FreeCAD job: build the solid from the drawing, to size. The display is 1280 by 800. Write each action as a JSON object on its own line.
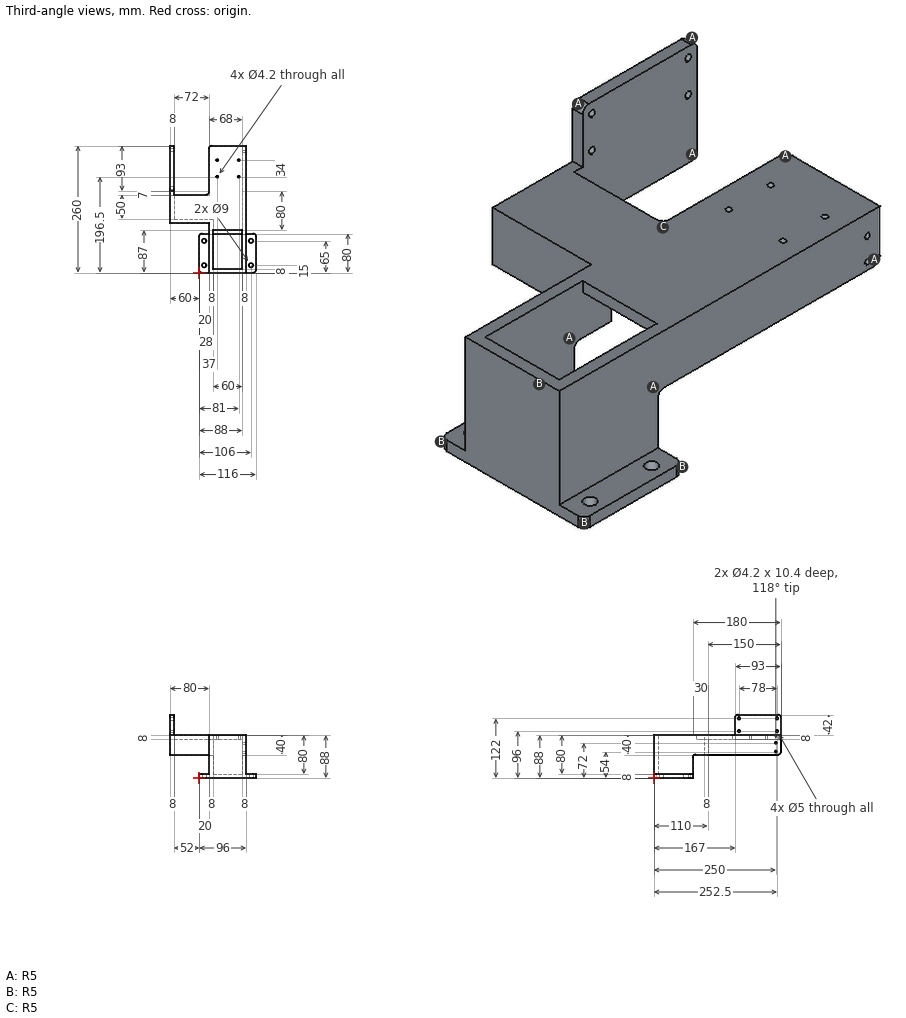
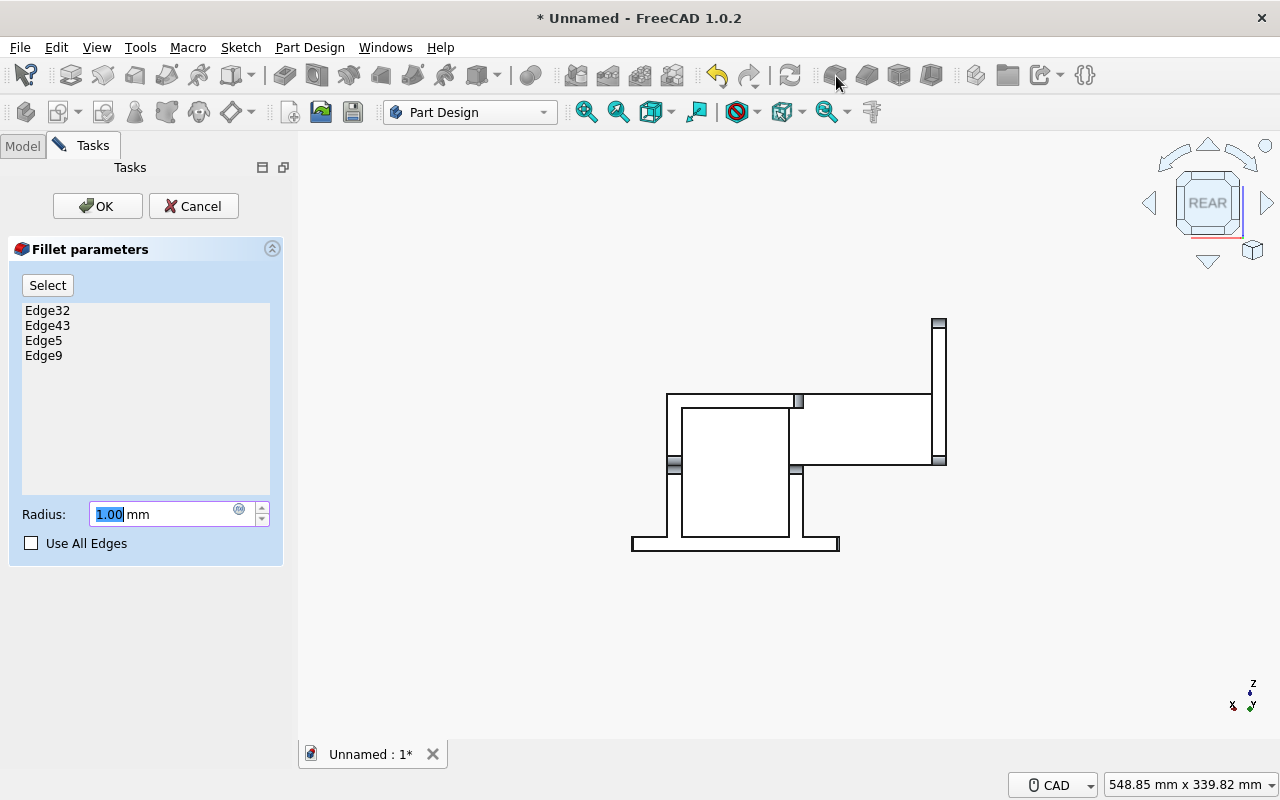
{"action": "type", "text": "5"}
{"action": "key", "text": "Tab"}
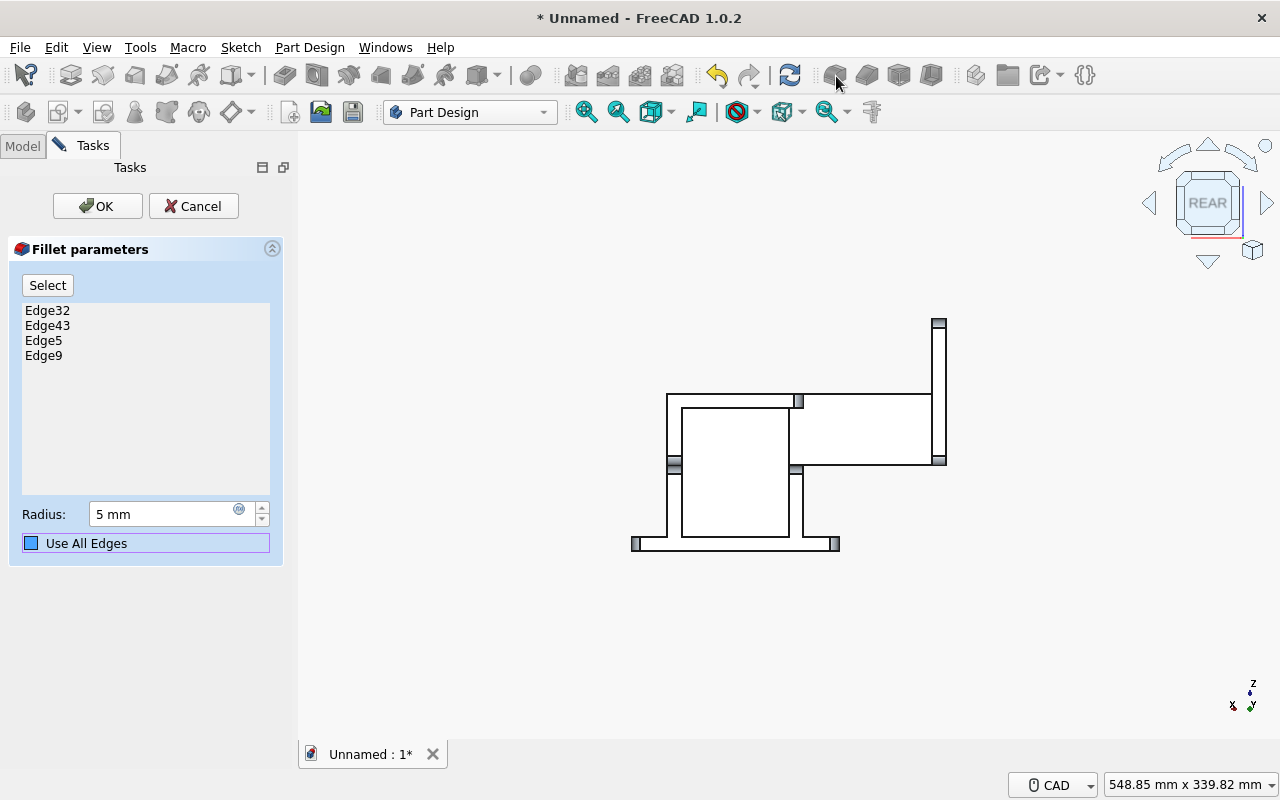
{"action": "left_click", "coordinate": [98, 206]}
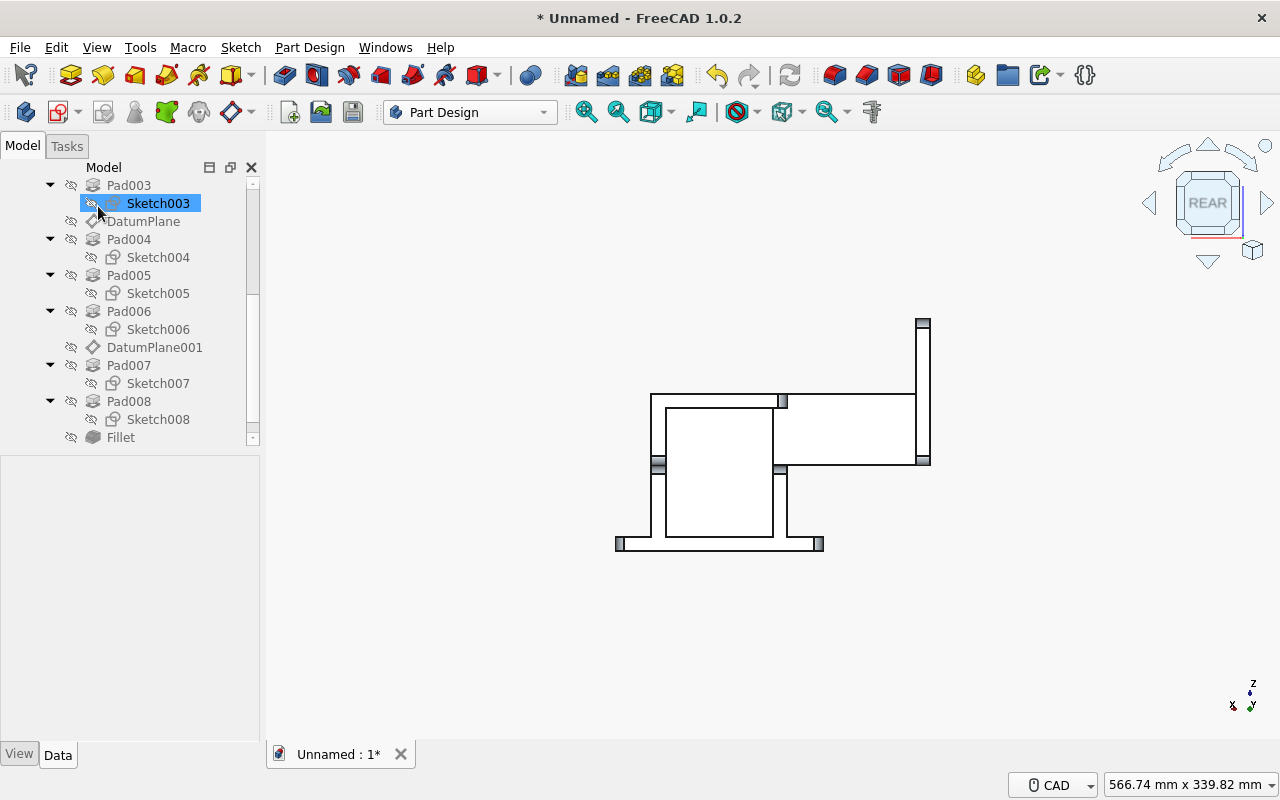
{"action": "left_click", "coordinate": [588, 112]}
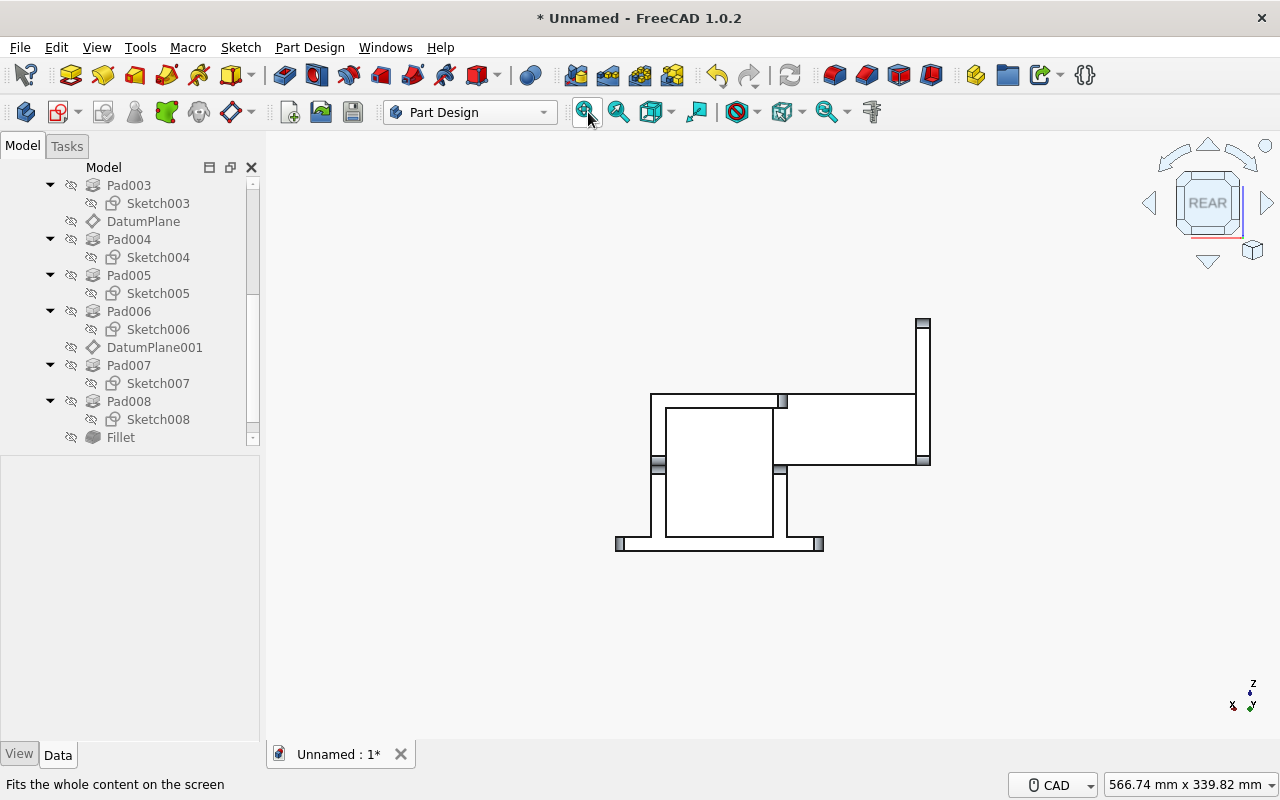
{"action": "key", "text": "0"}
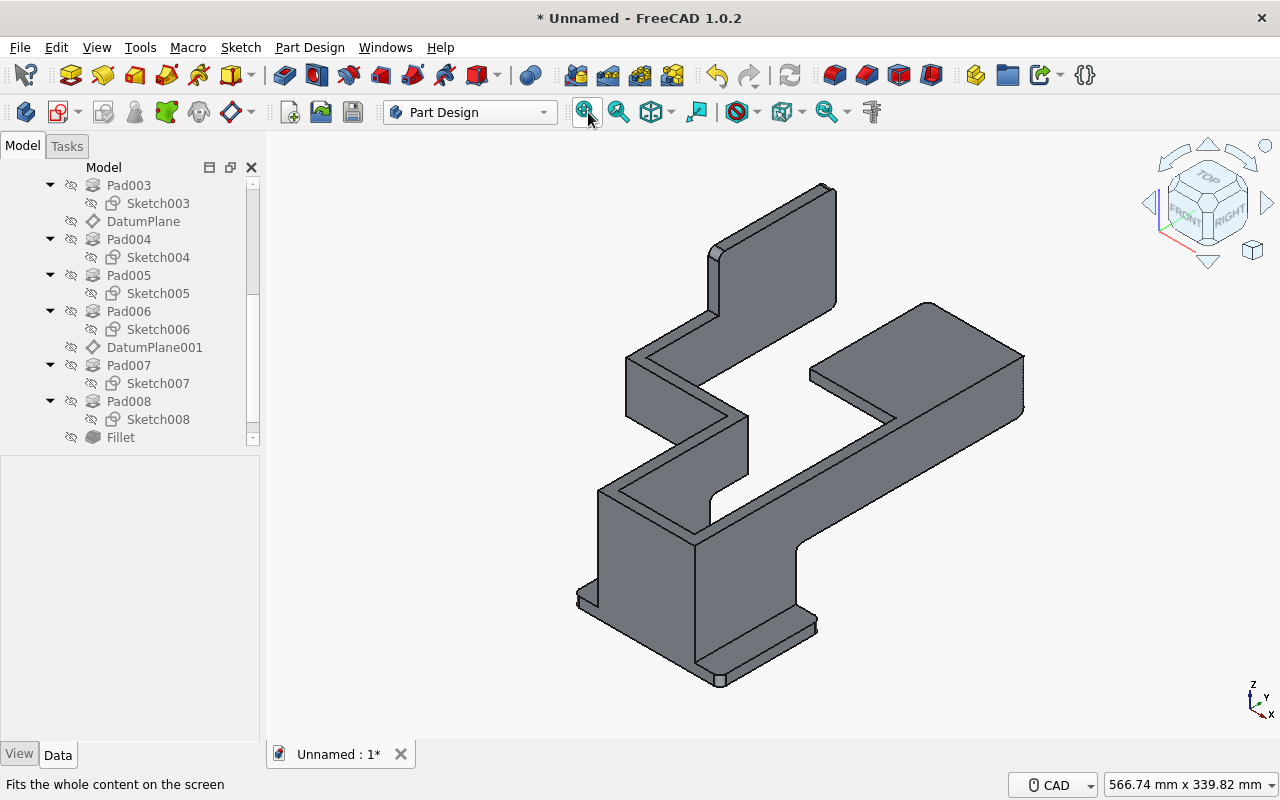
{"action": "key", "text": "2"}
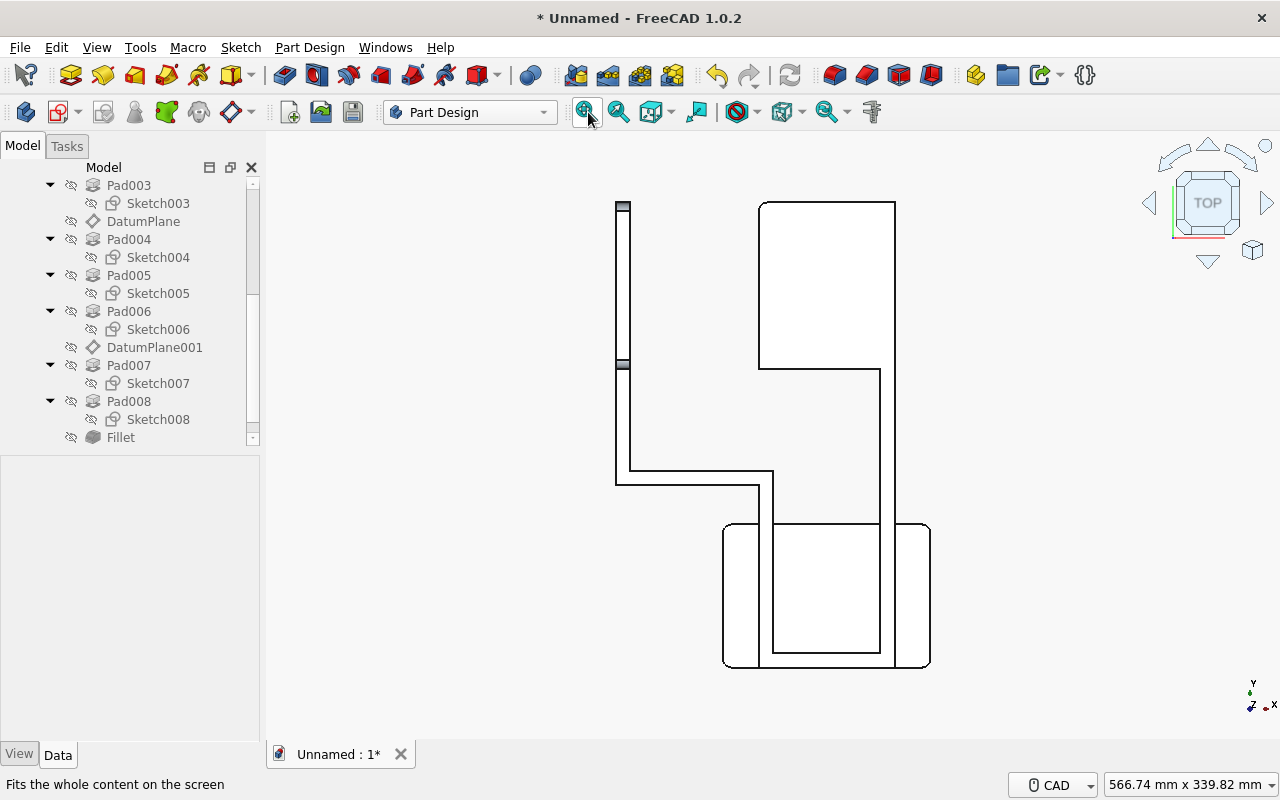
{"action": "left_click", "coordinate": [827, 588]}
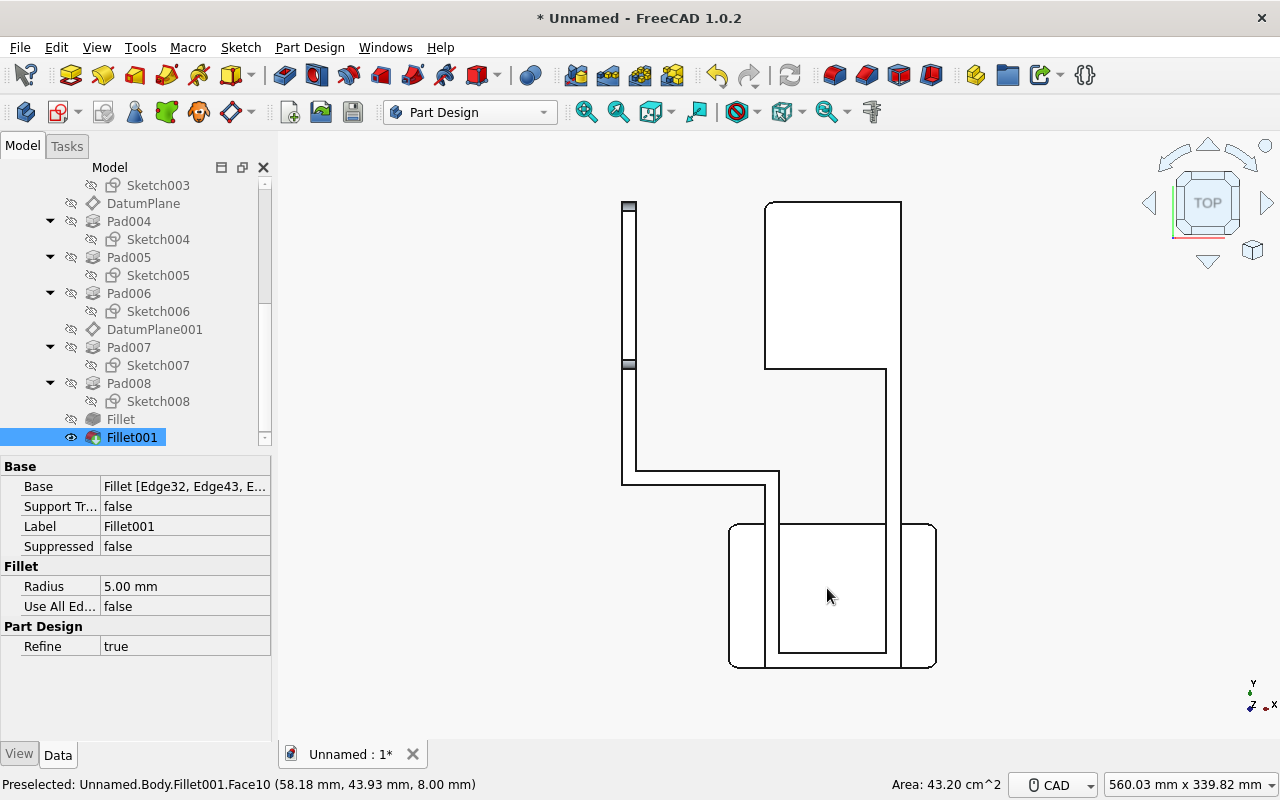
{"action": "left_click", "coordinate": [58, 112]}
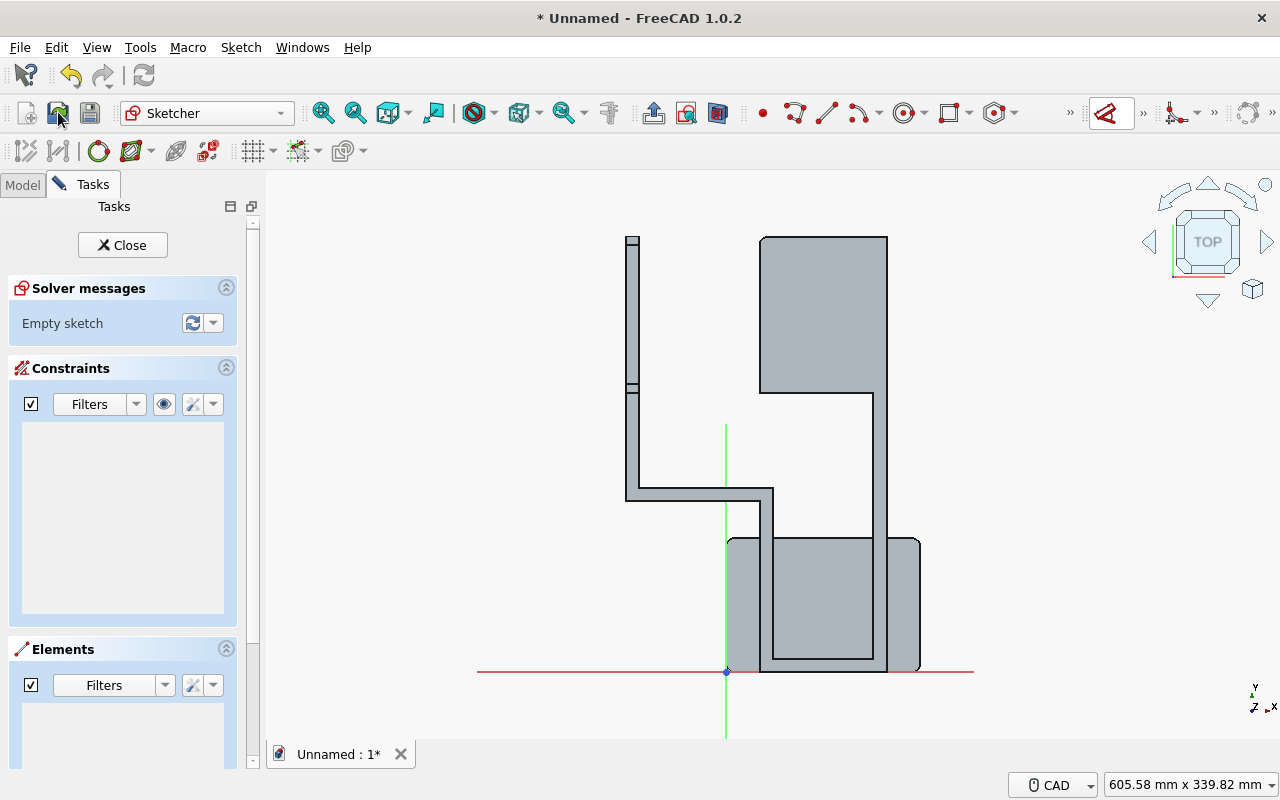
{"action": "left_click", "coordinate": [718, 114]}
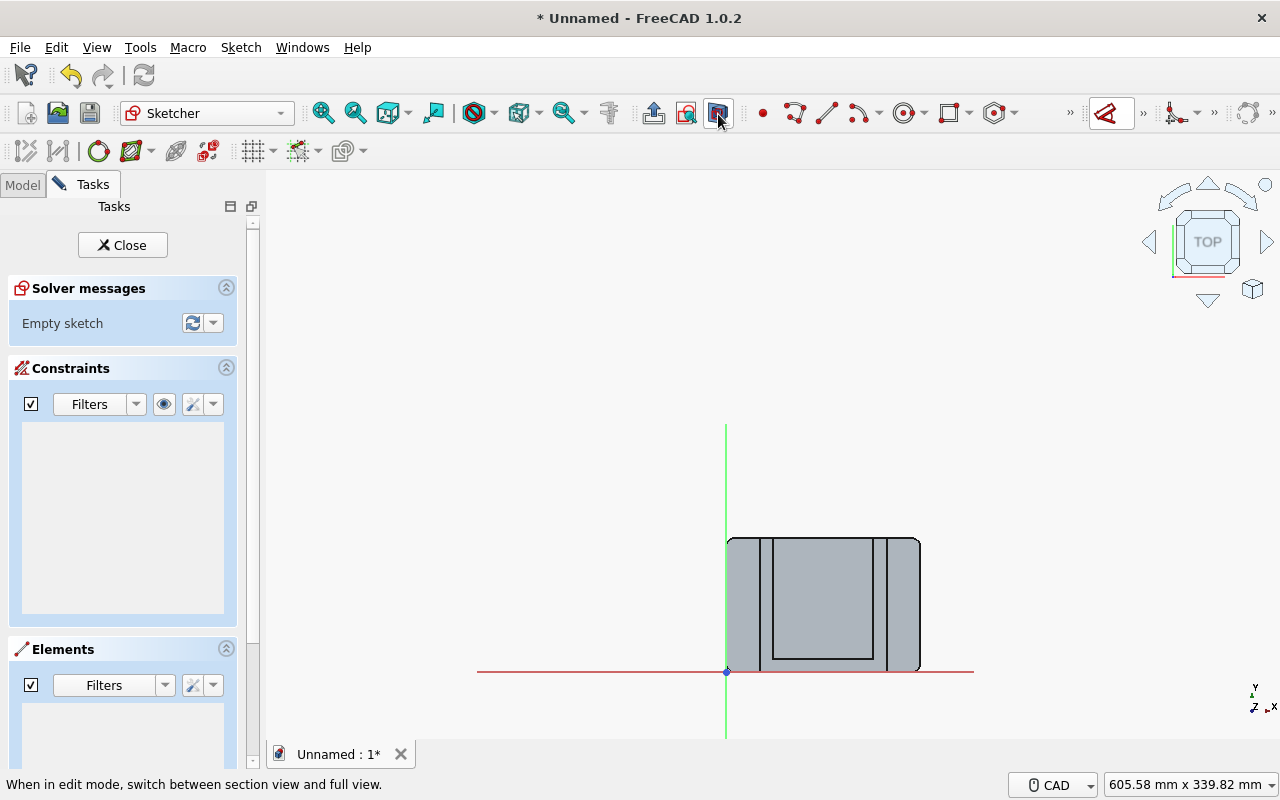
{"action": "scroll", "coordinate": [868, 683], "scroll_direction": "up", "scroll_amount": 6}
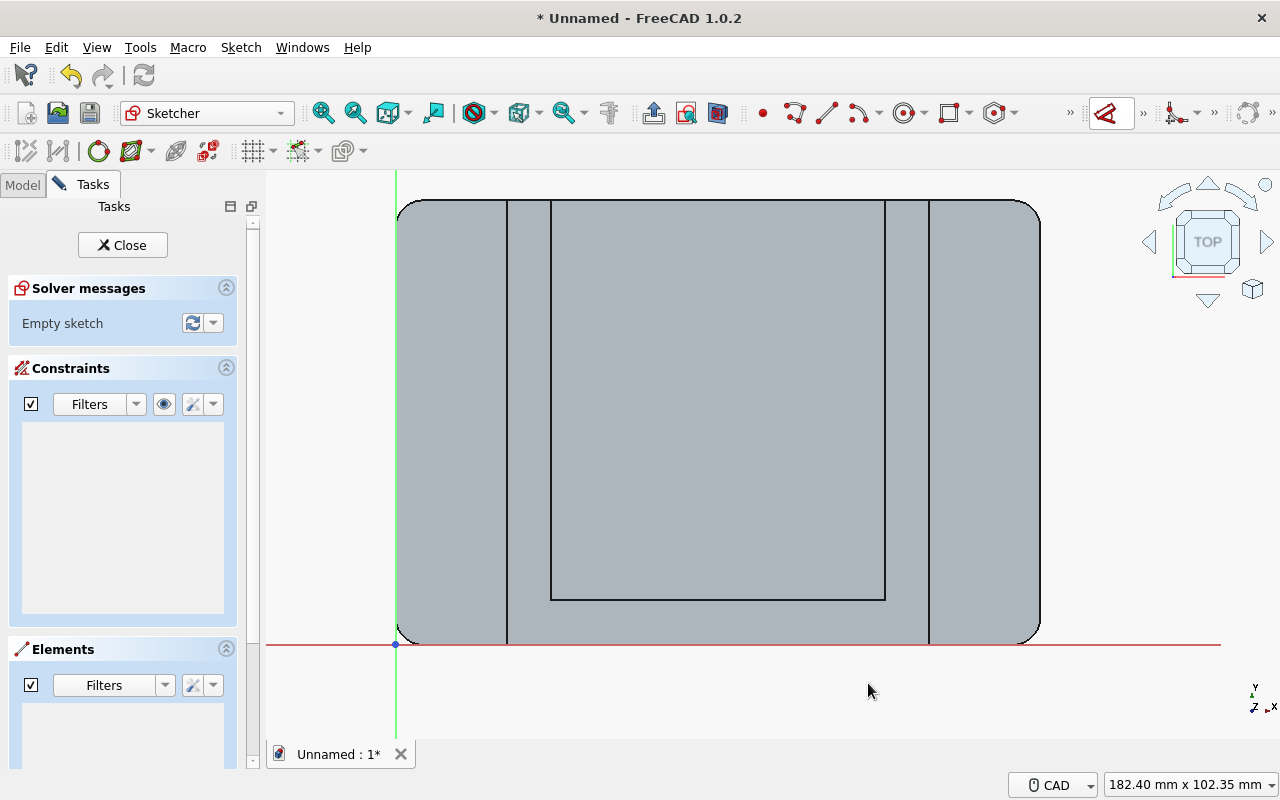
{"action": "left_click", "coordinate": [904, 114]}